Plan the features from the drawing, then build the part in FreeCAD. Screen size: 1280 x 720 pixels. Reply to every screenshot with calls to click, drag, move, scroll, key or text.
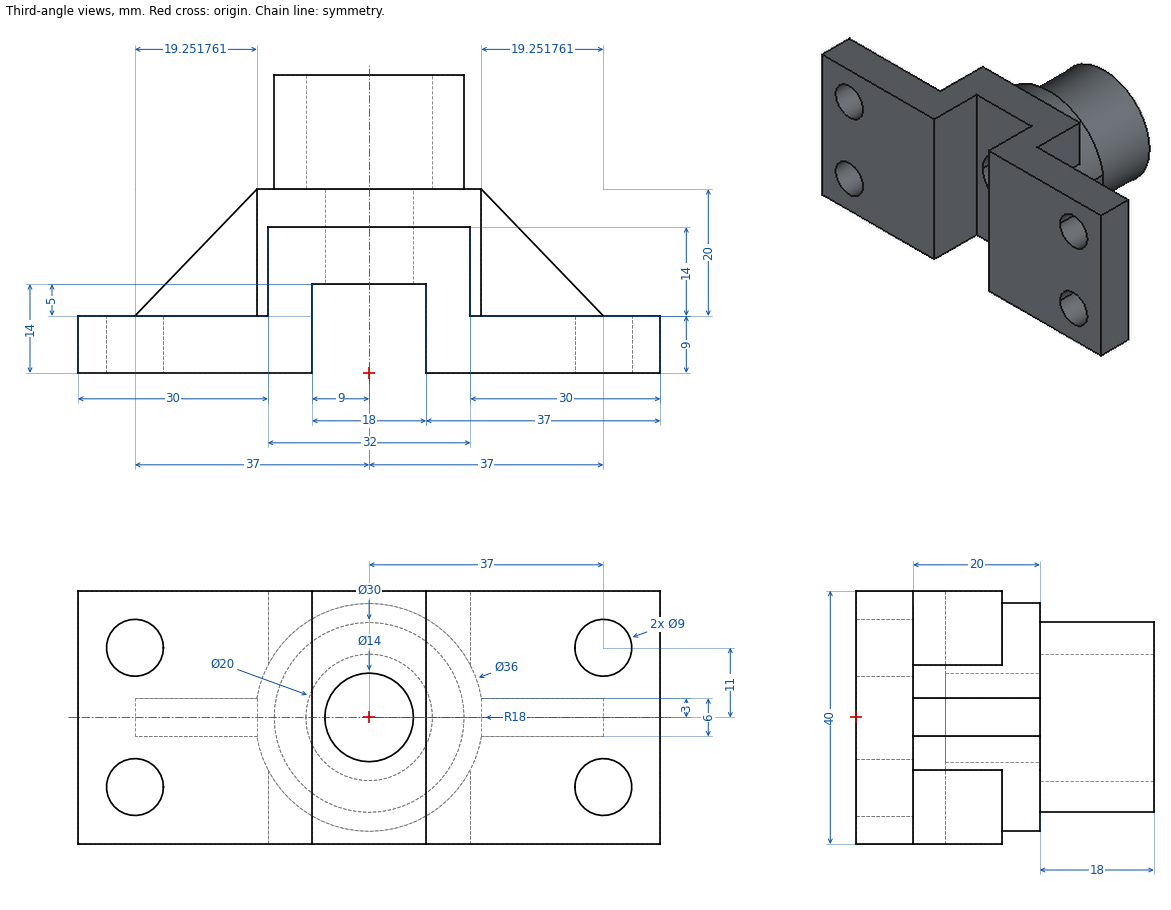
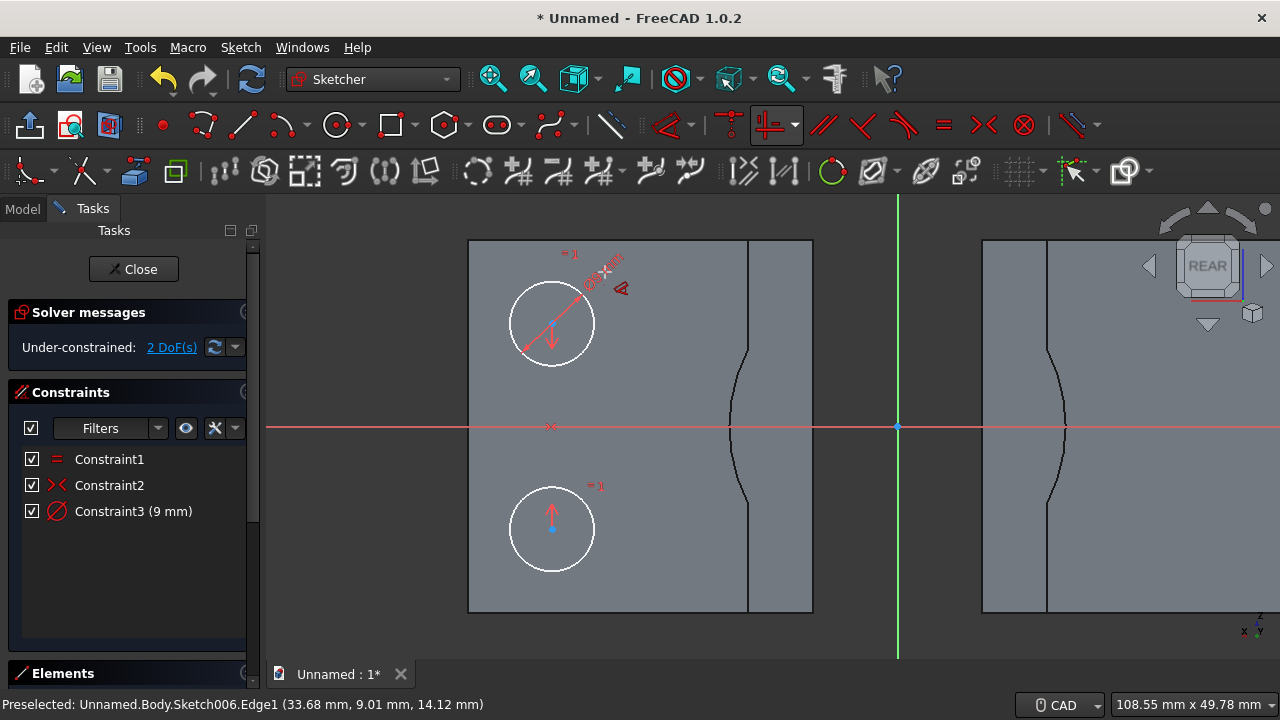
click(552, 324)
click(725, 290)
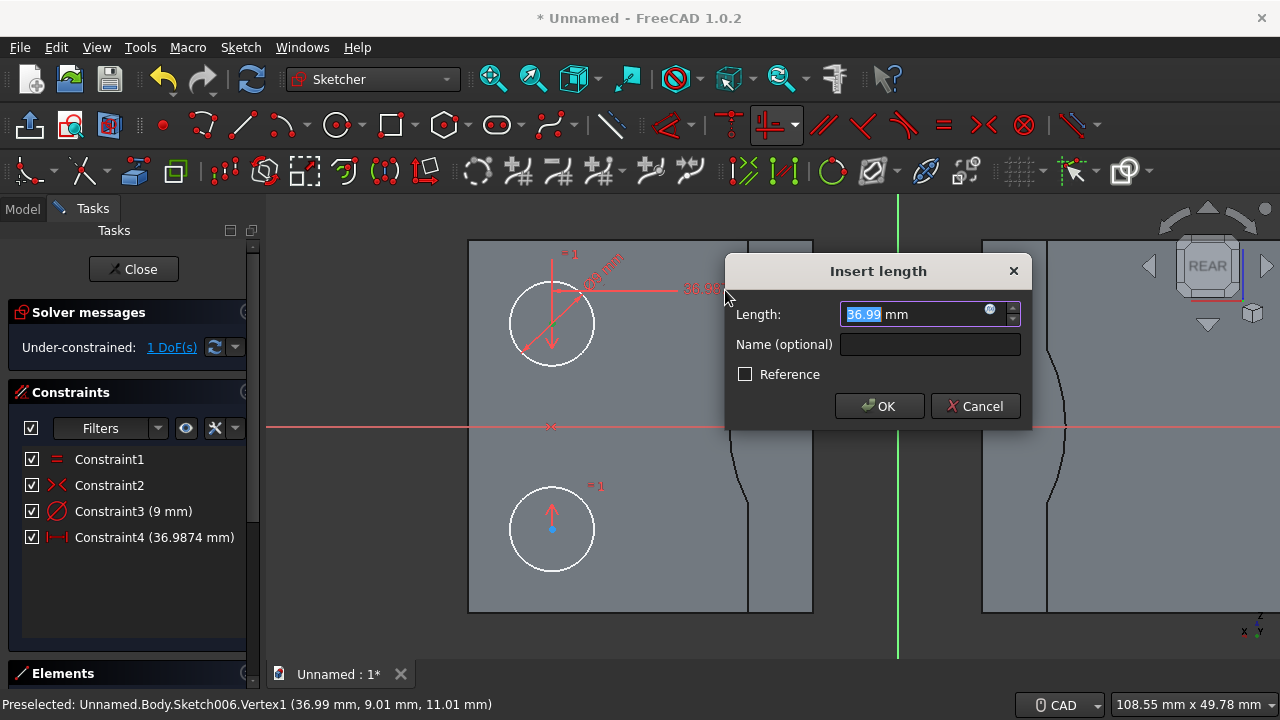
text(37)
key(Return)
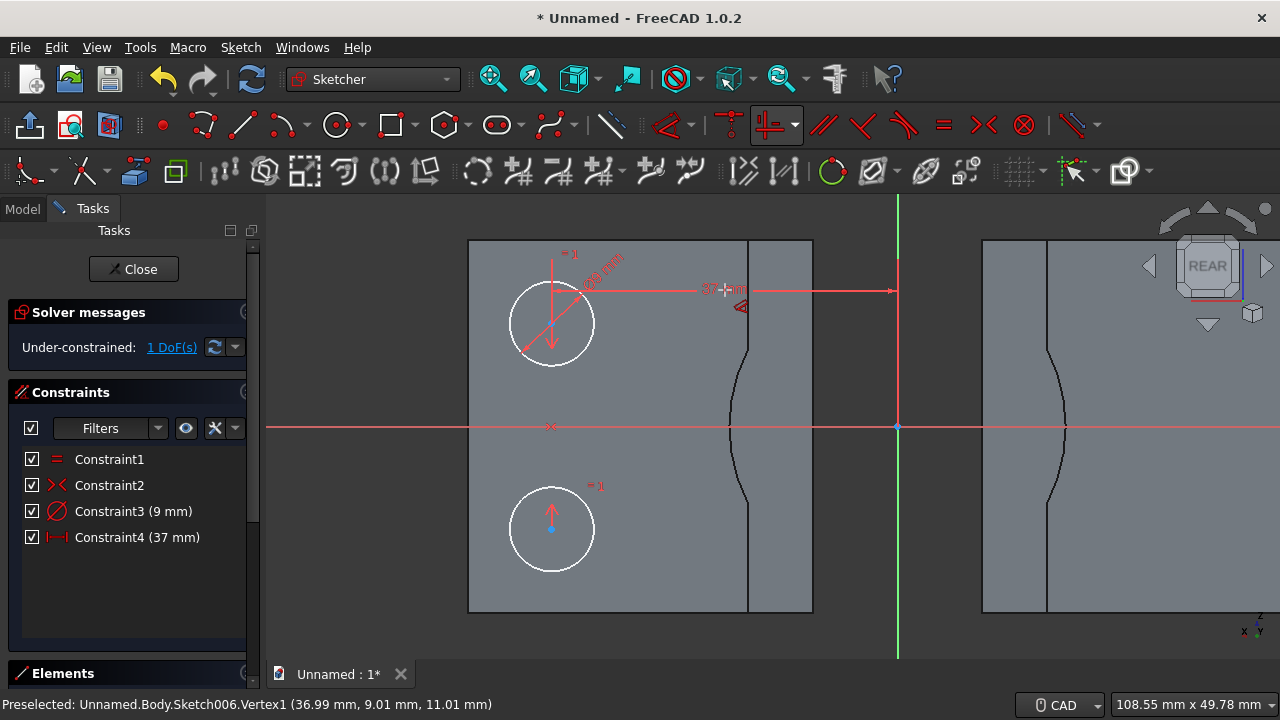
click(552, 324)
click(932, 375)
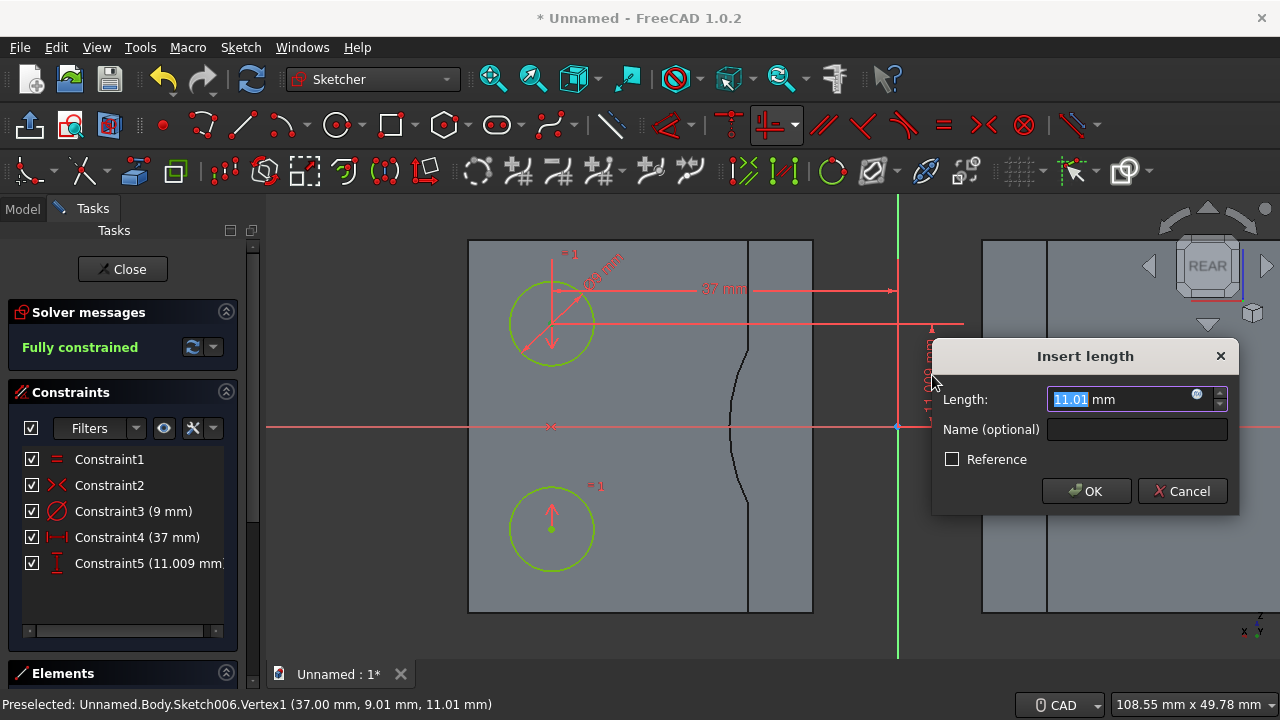
text(11)
key(Return)
key(Escape)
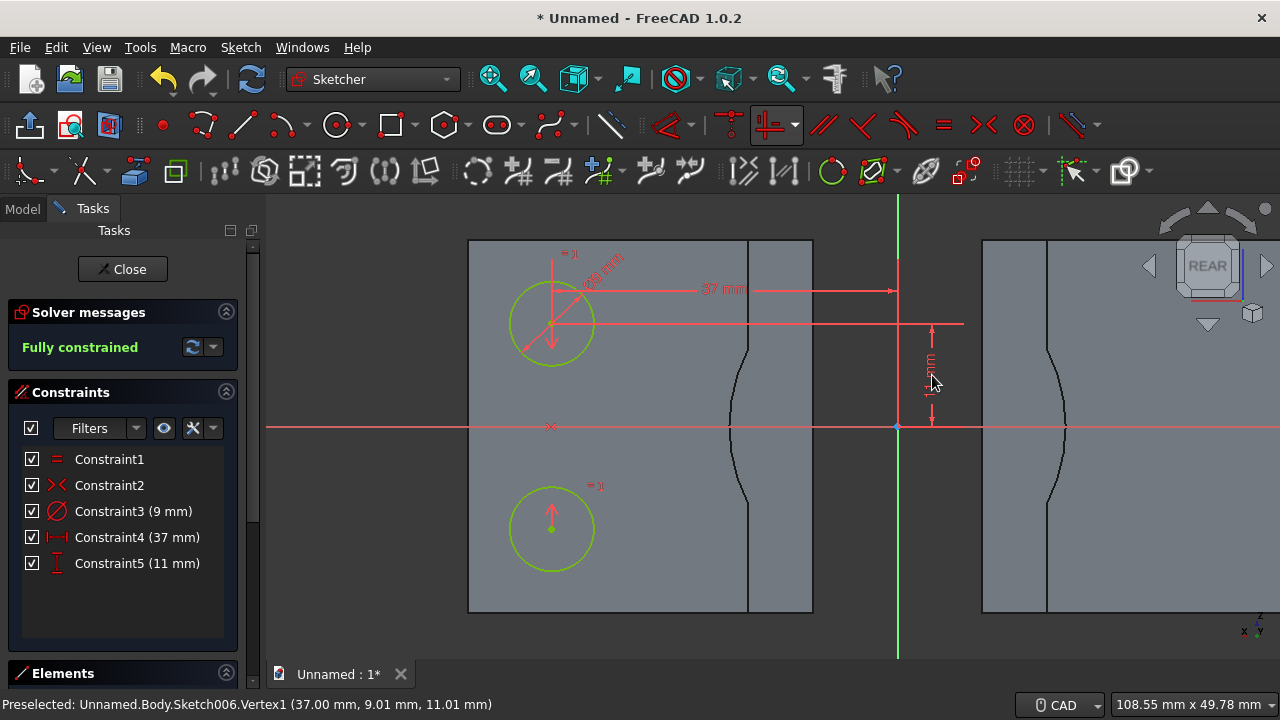
click(123, 269)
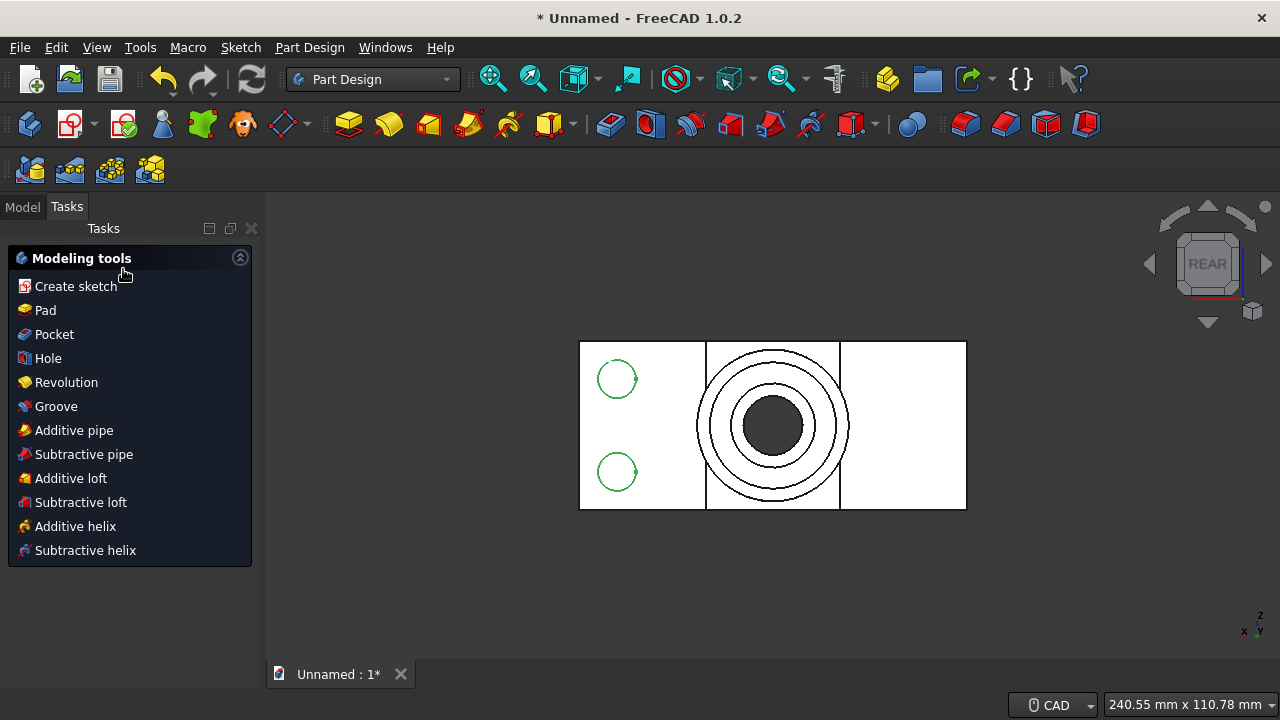
click(612, 124)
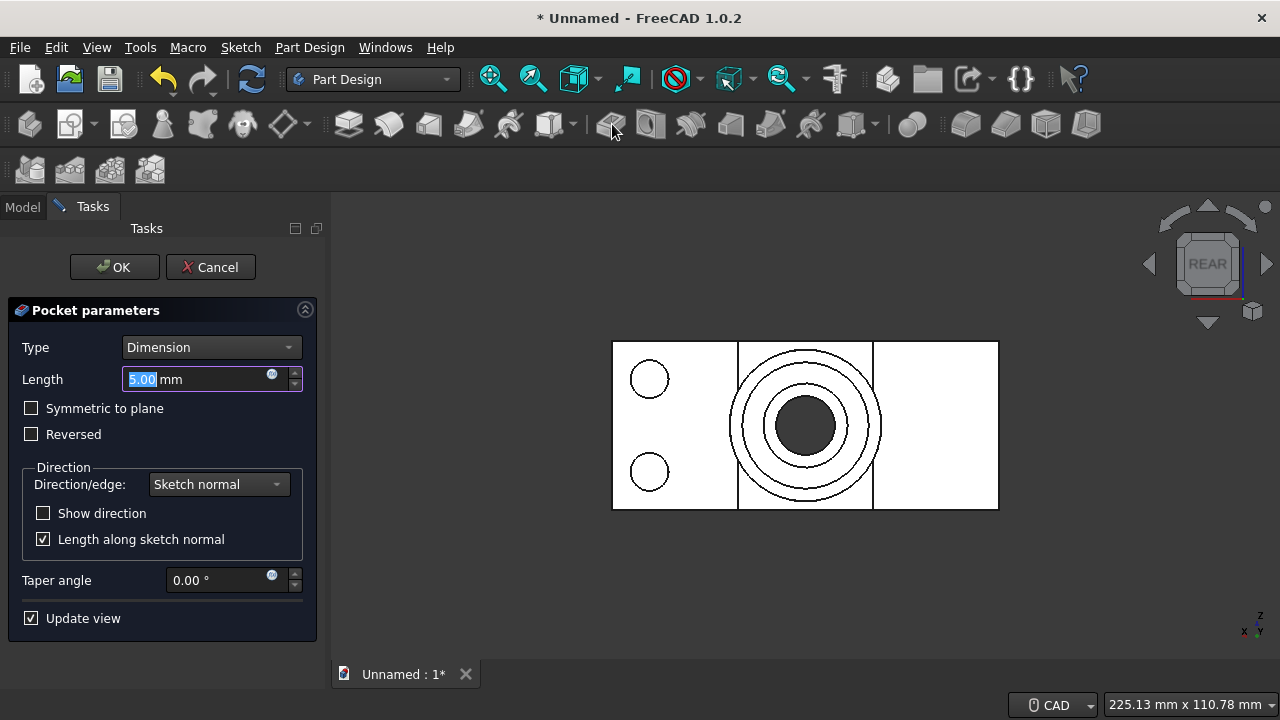
click(212, 348)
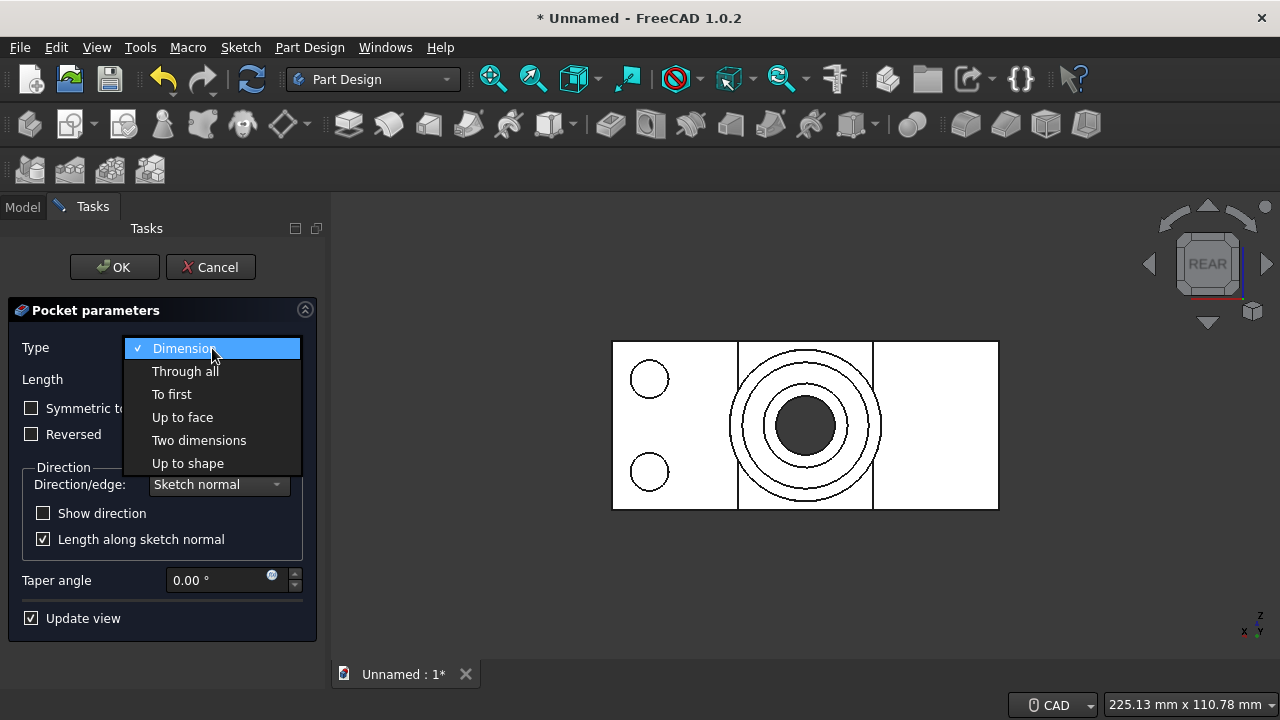
click(212, 372)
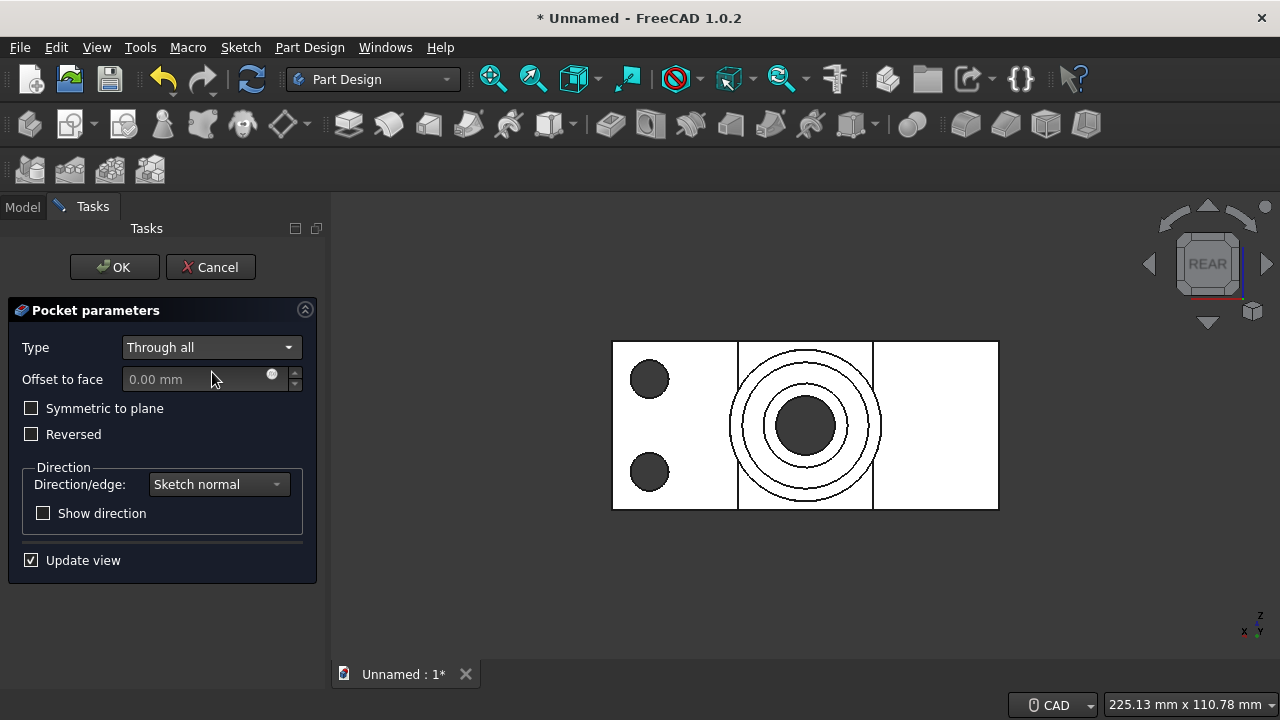
click(115, 267)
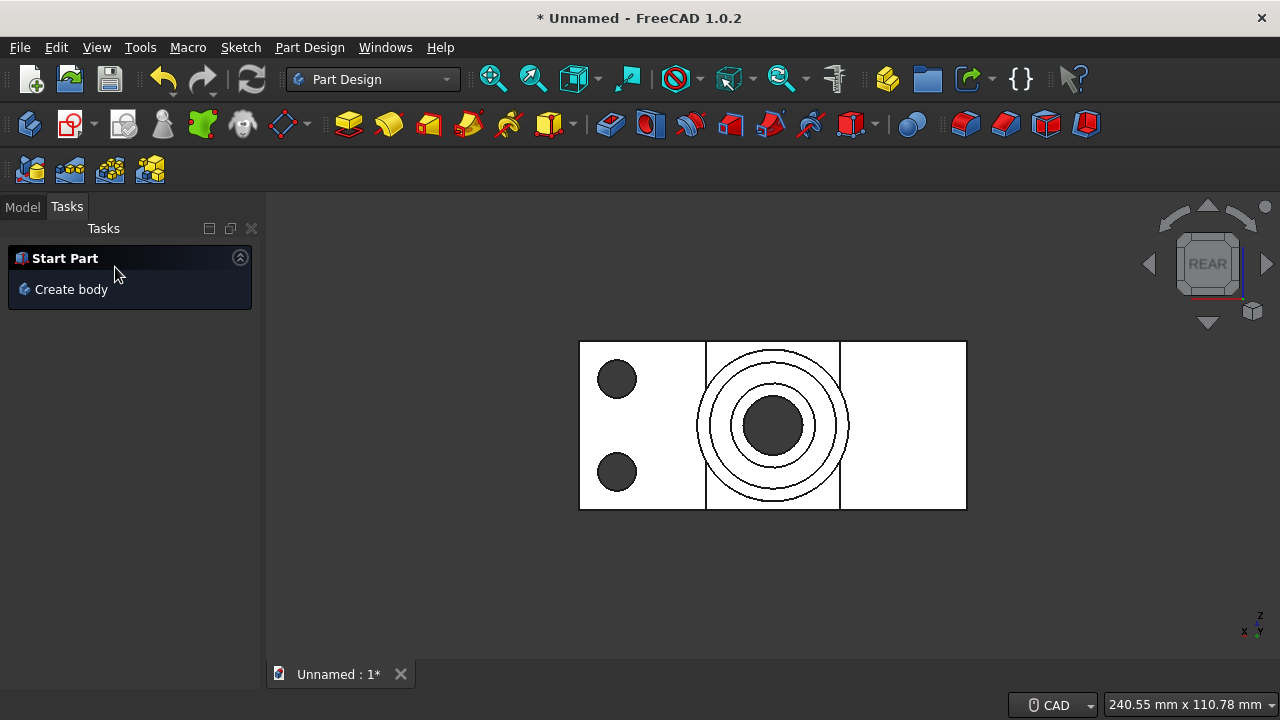
key(v)
key(f)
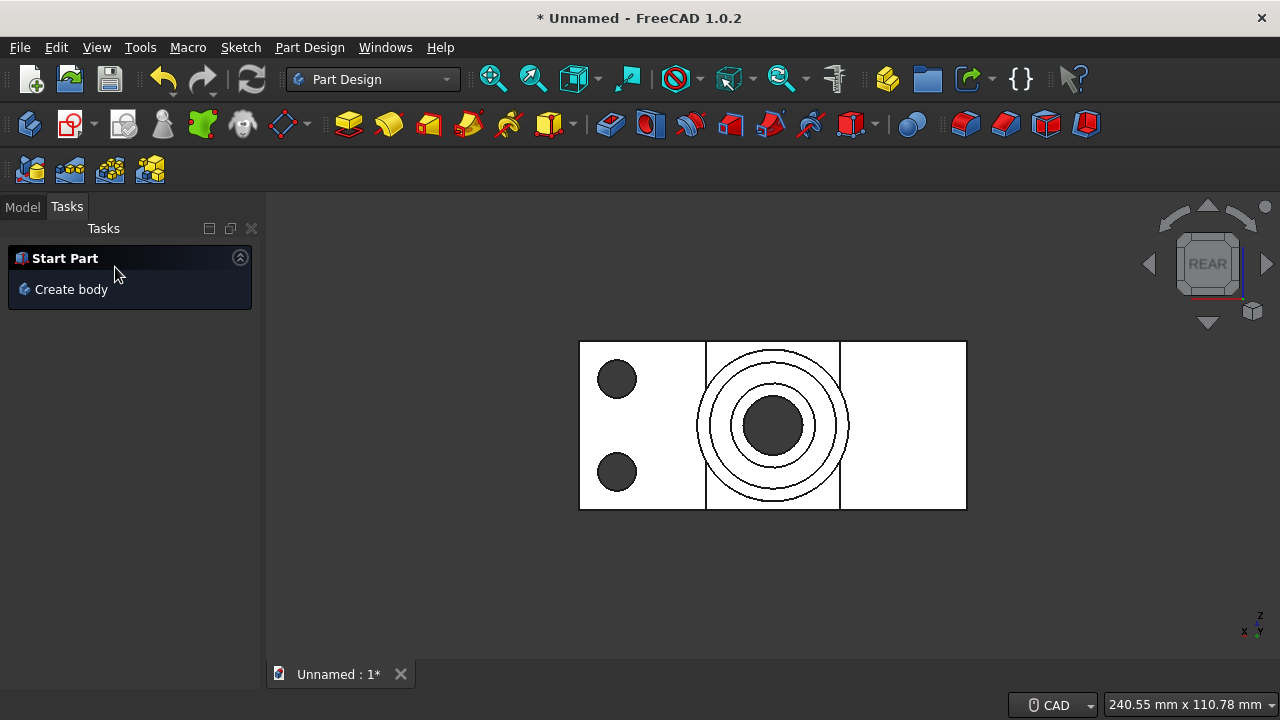
click(904, 400)